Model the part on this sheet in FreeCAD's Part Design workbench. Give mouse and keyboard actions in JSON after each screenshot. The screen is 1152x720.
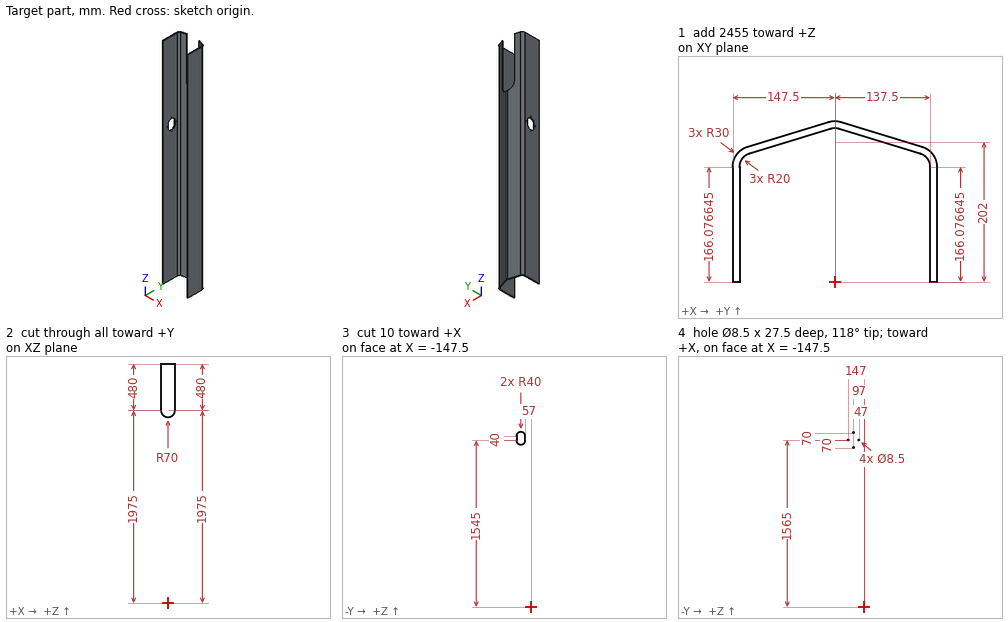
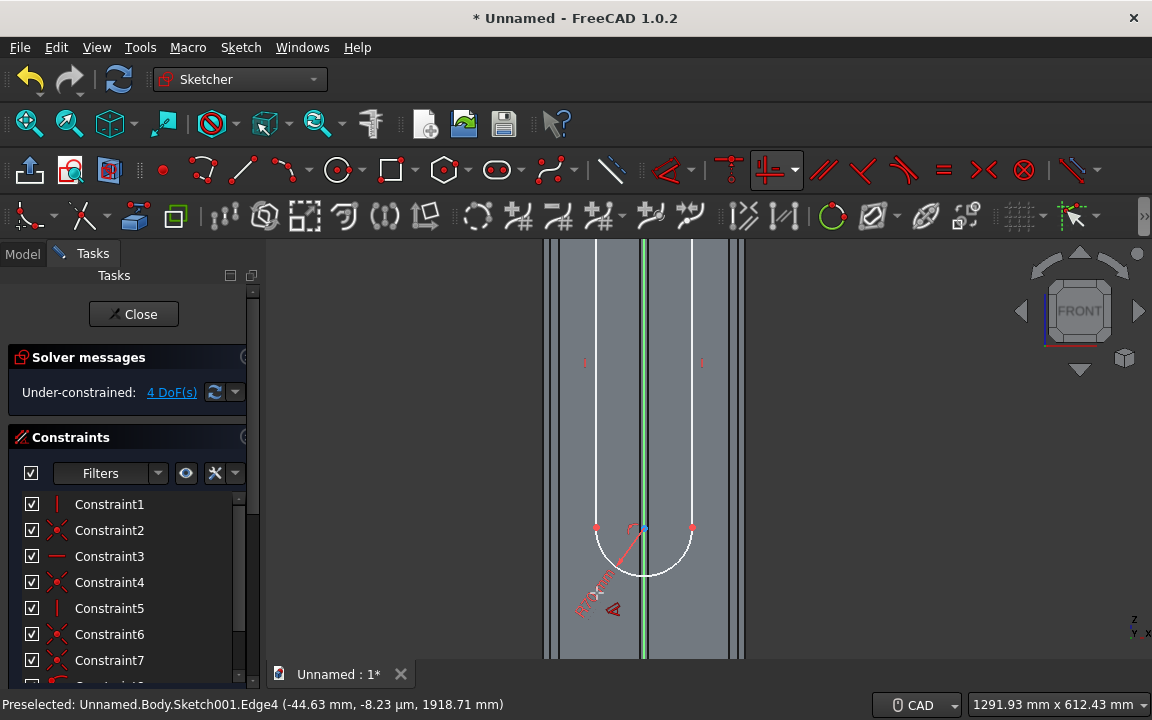
{"action": "left_click", "coordinate": [596, 429]}
{"action": "left_click", "coordinate": [562, 397]}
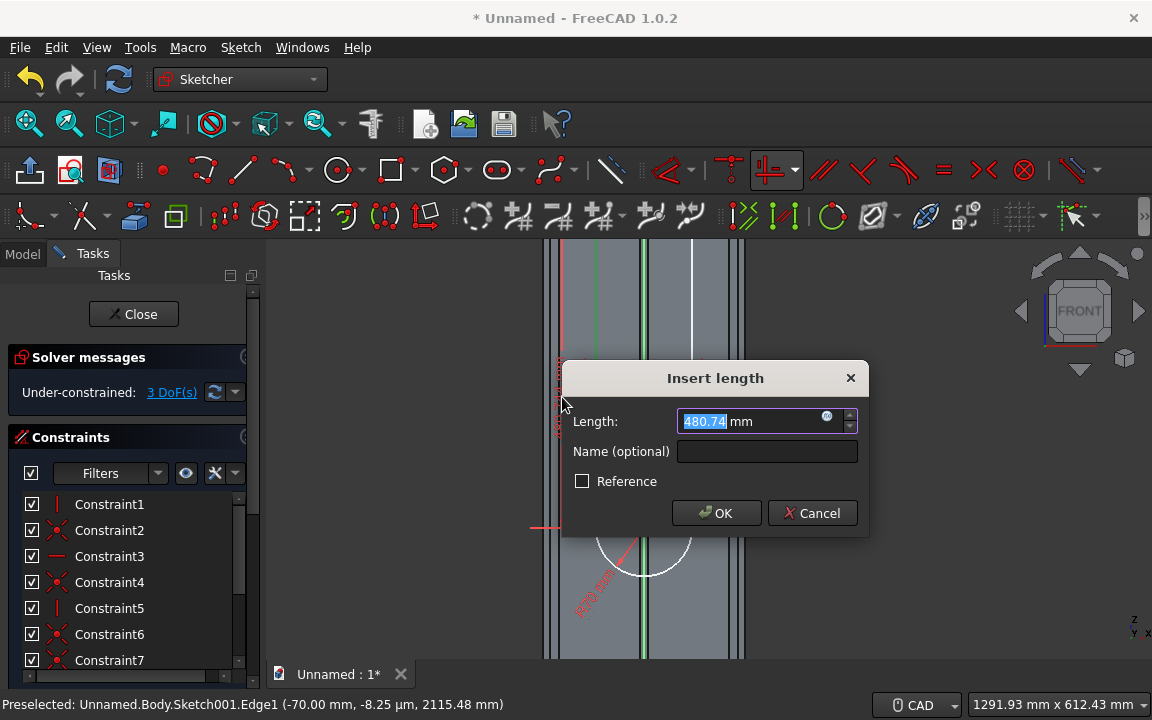
{"action": "type", "text": "480"}
{"action": "key", "text": "Return"}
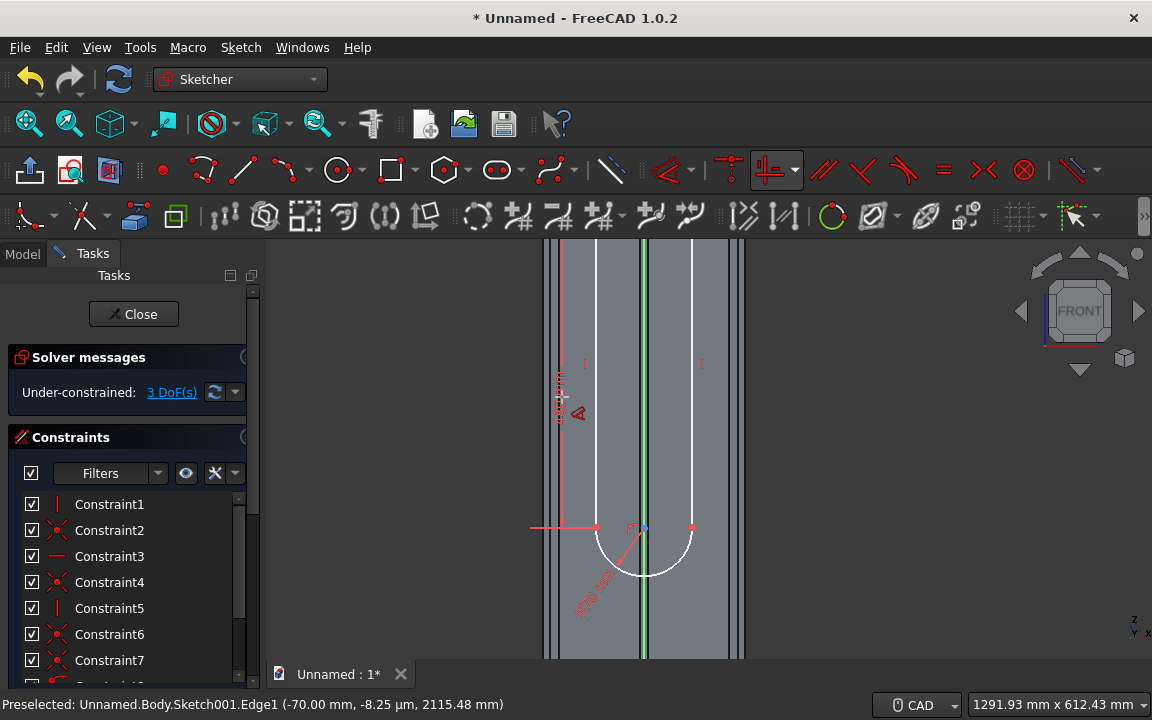
{"action": "left_click", "coordinate": [692, 297]}
{"action": "left_click", "coordinate": [726, 397]}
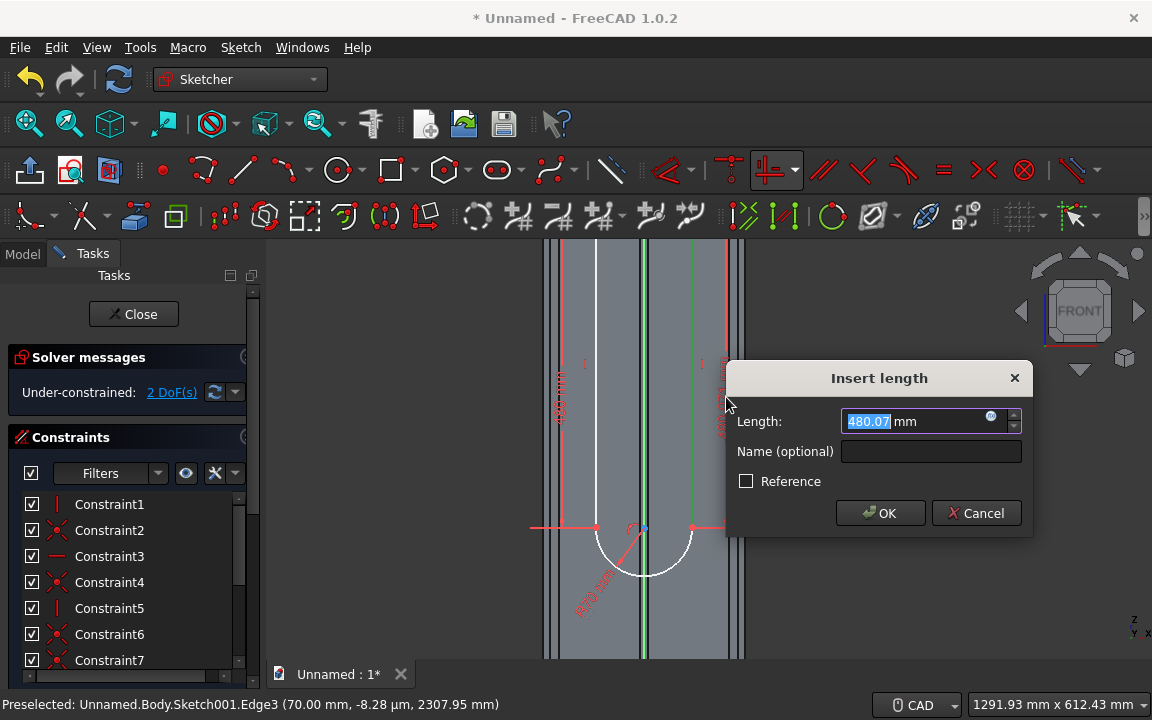
{"action": "type", "text": "480"}
{"action": "key", "text": "Return"}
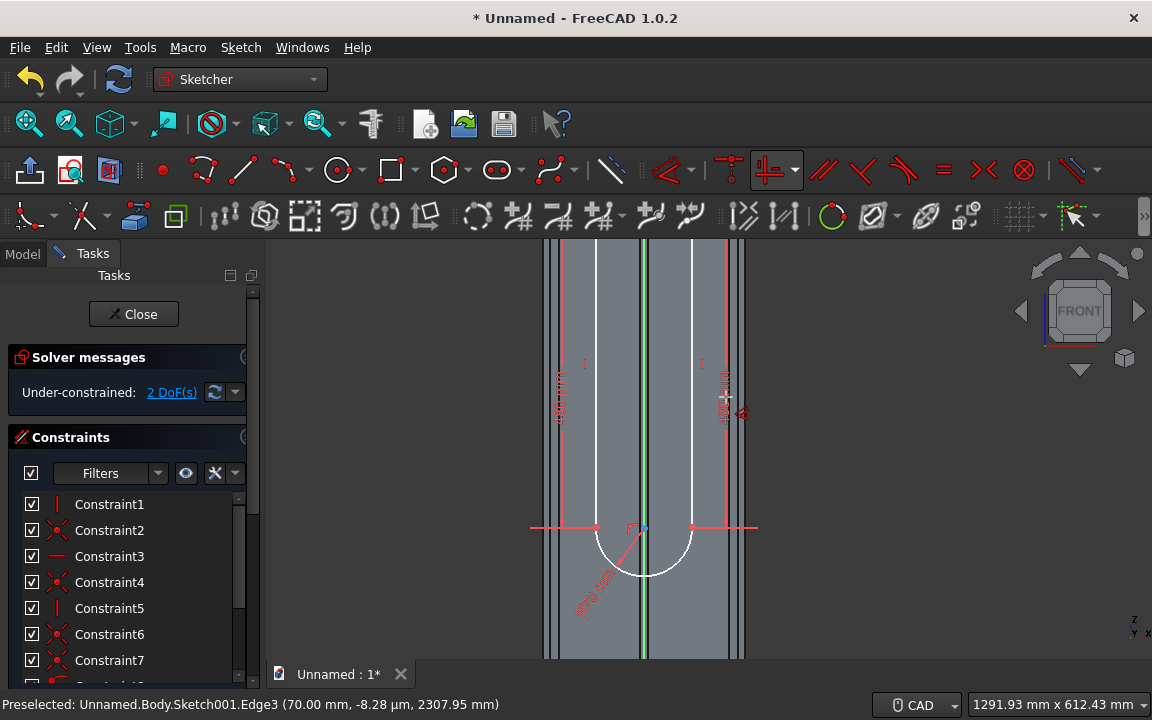
{"action": "left_click", "coordinate": [596, 528]}
{"action": "left_click", "coordinate": [562, 556]}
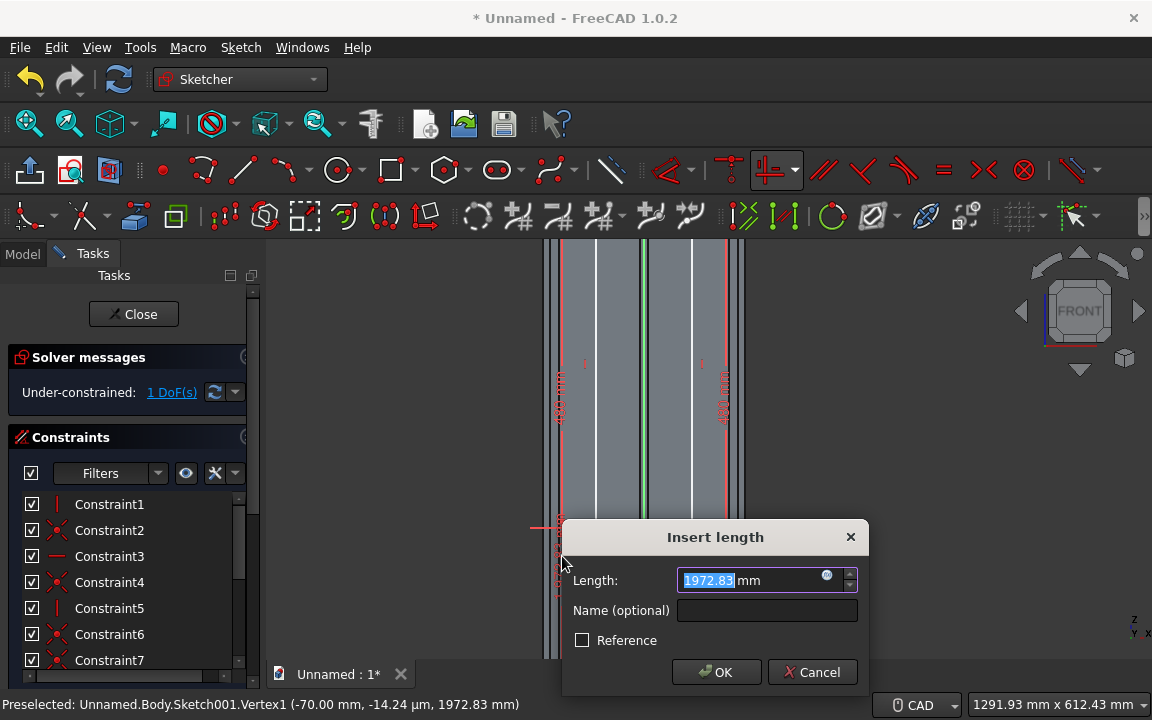
{"action": "type", "text": "1975"}
{"action": "key", "text": "Return"}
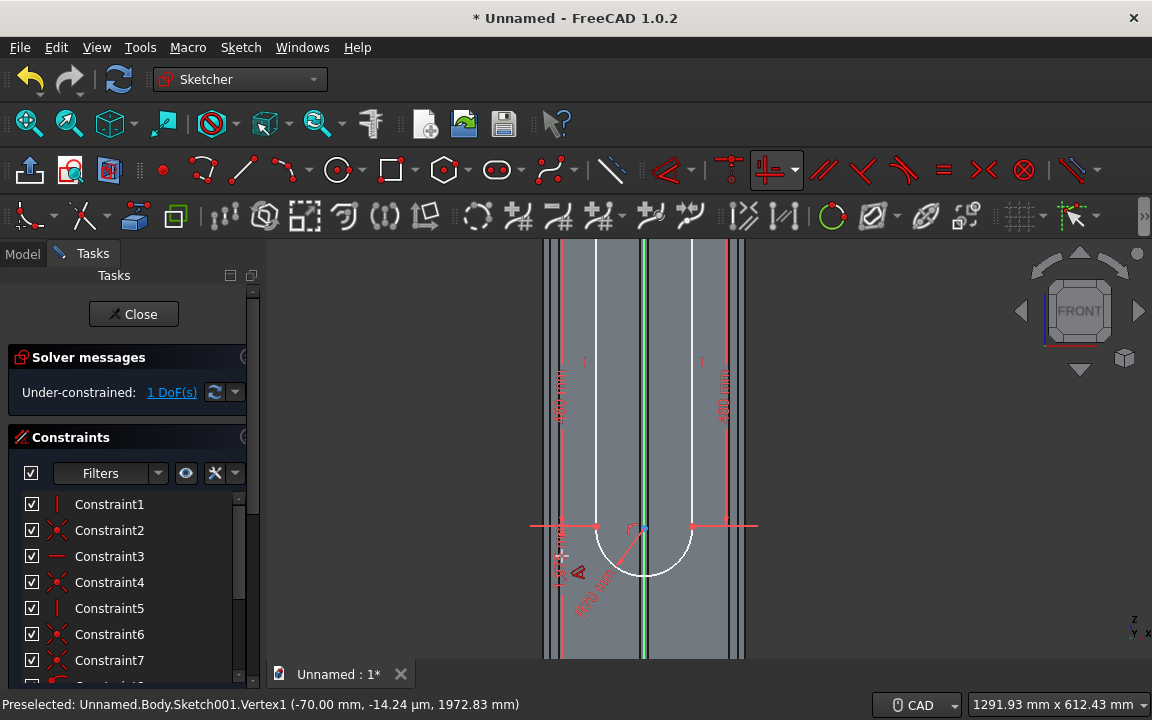
{"action": "left_click", "coordinate": [644, 528]}
{"action": "left_click", "coordinate": [678, 580]}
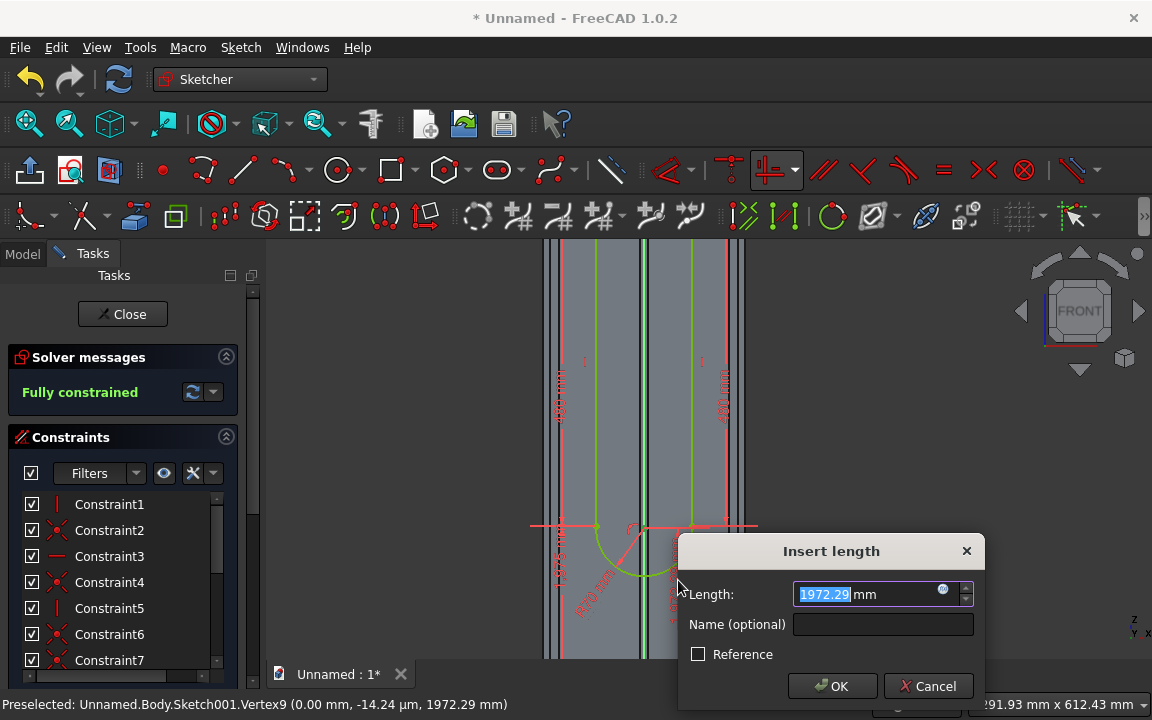
{"action": "type", "text": "1975"}
{"action": "key", "text": "Return"}
{"action": "key", "text": "Escape"}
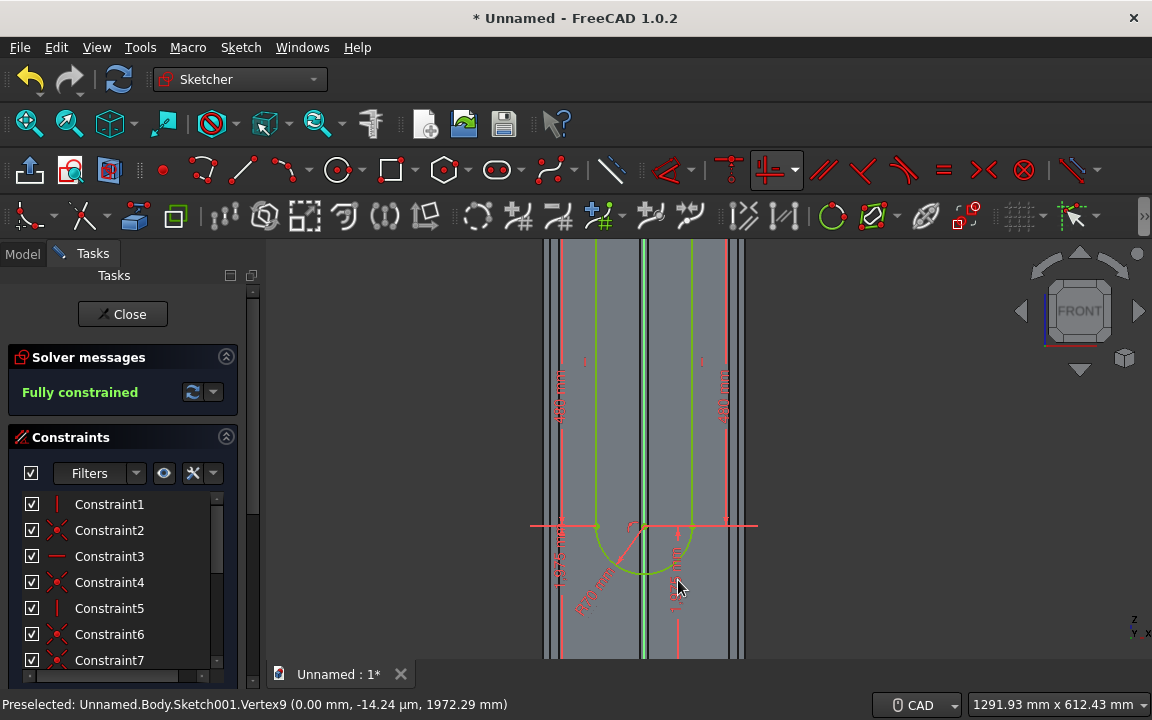
{"action": "left_click", "coordinate": [123, 314]}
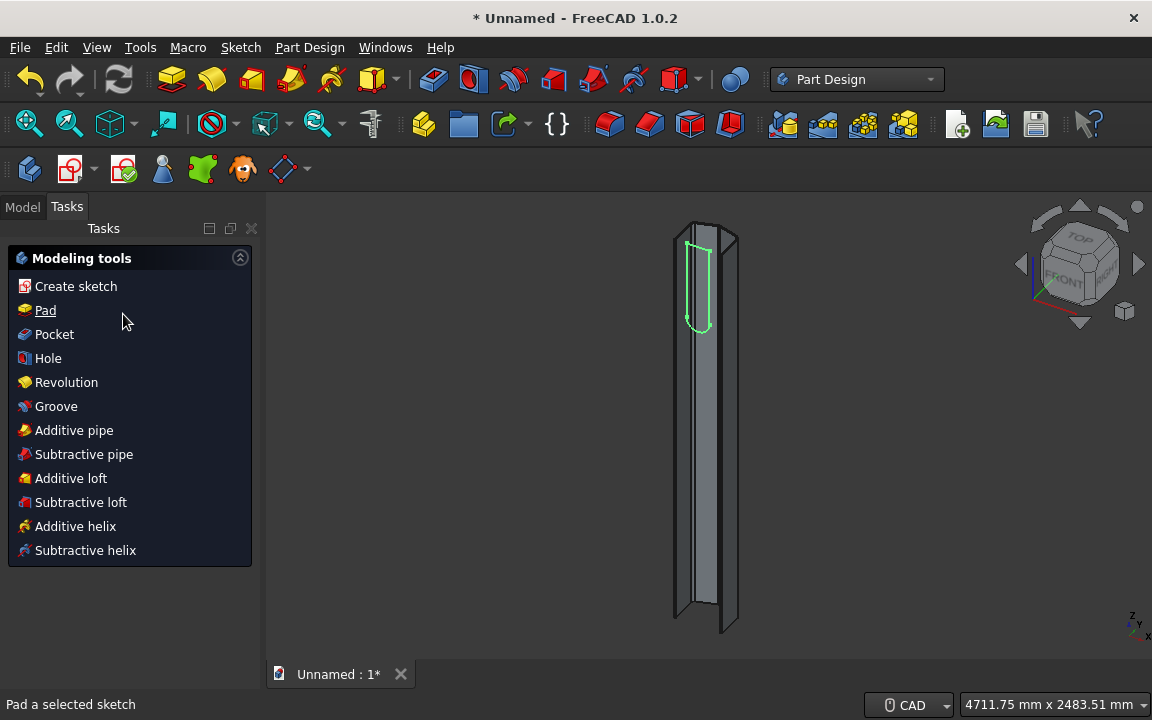
{"action": "left_click", "coordinate": [434, 80]}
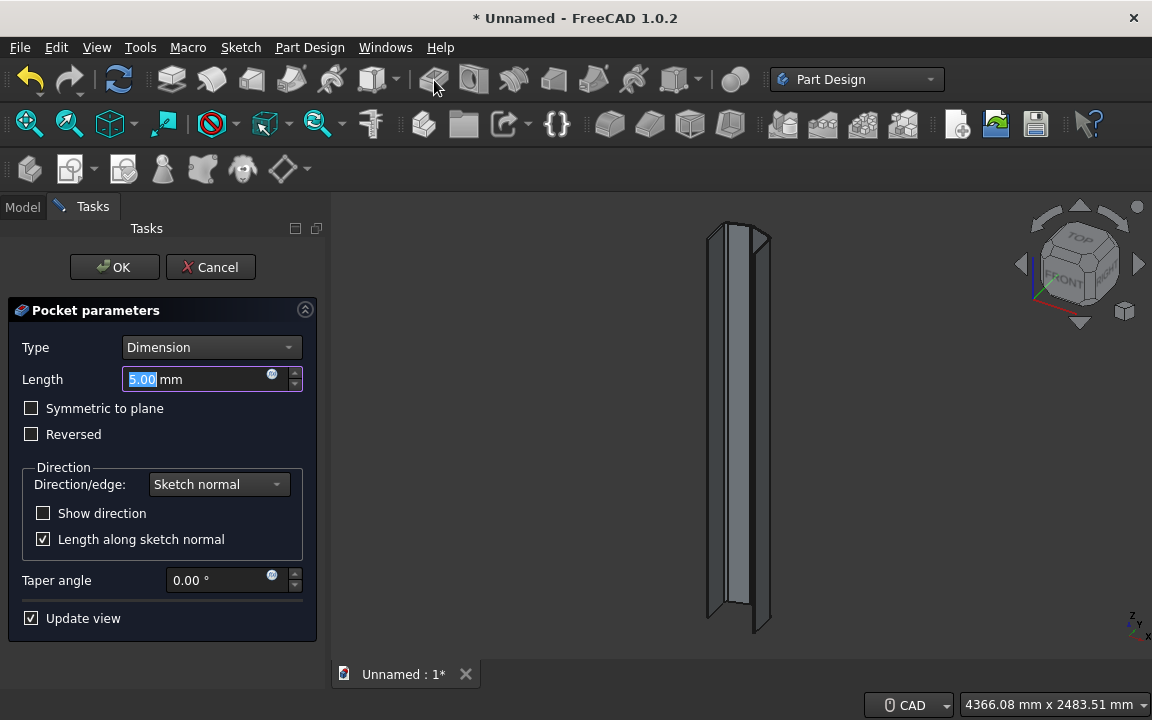
{"action": "left_click", "coordinate": [212, 348]}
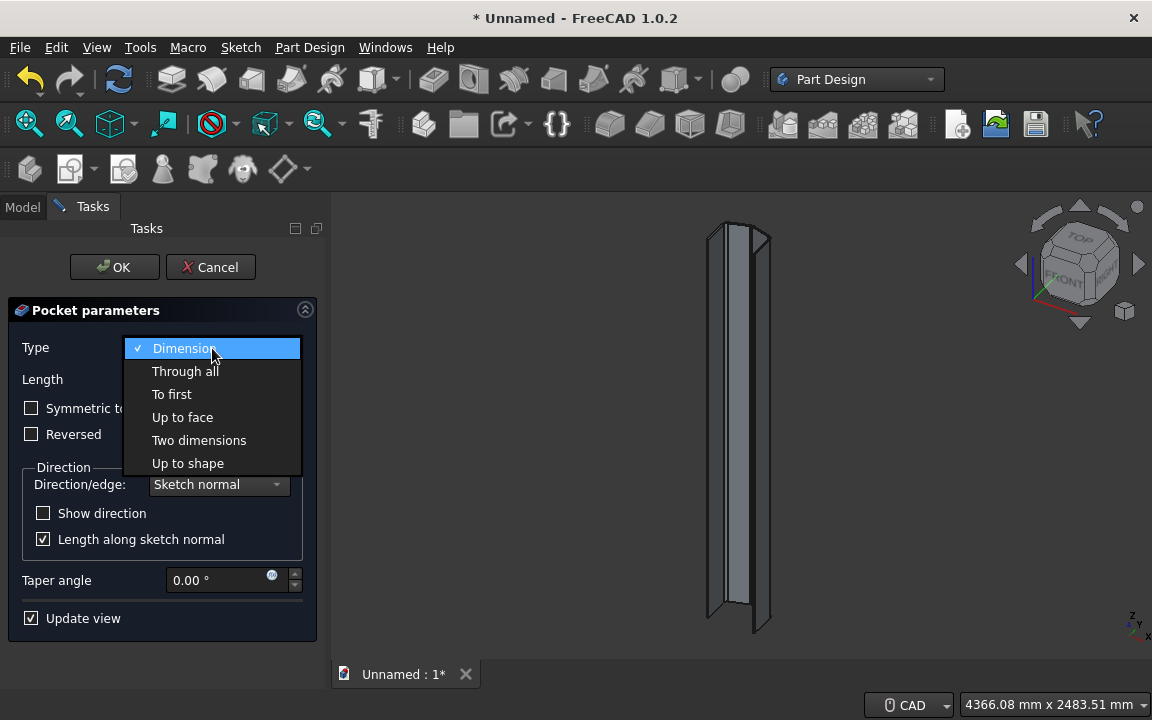
{"action": "left_click", "coordinate": [212, 372]}